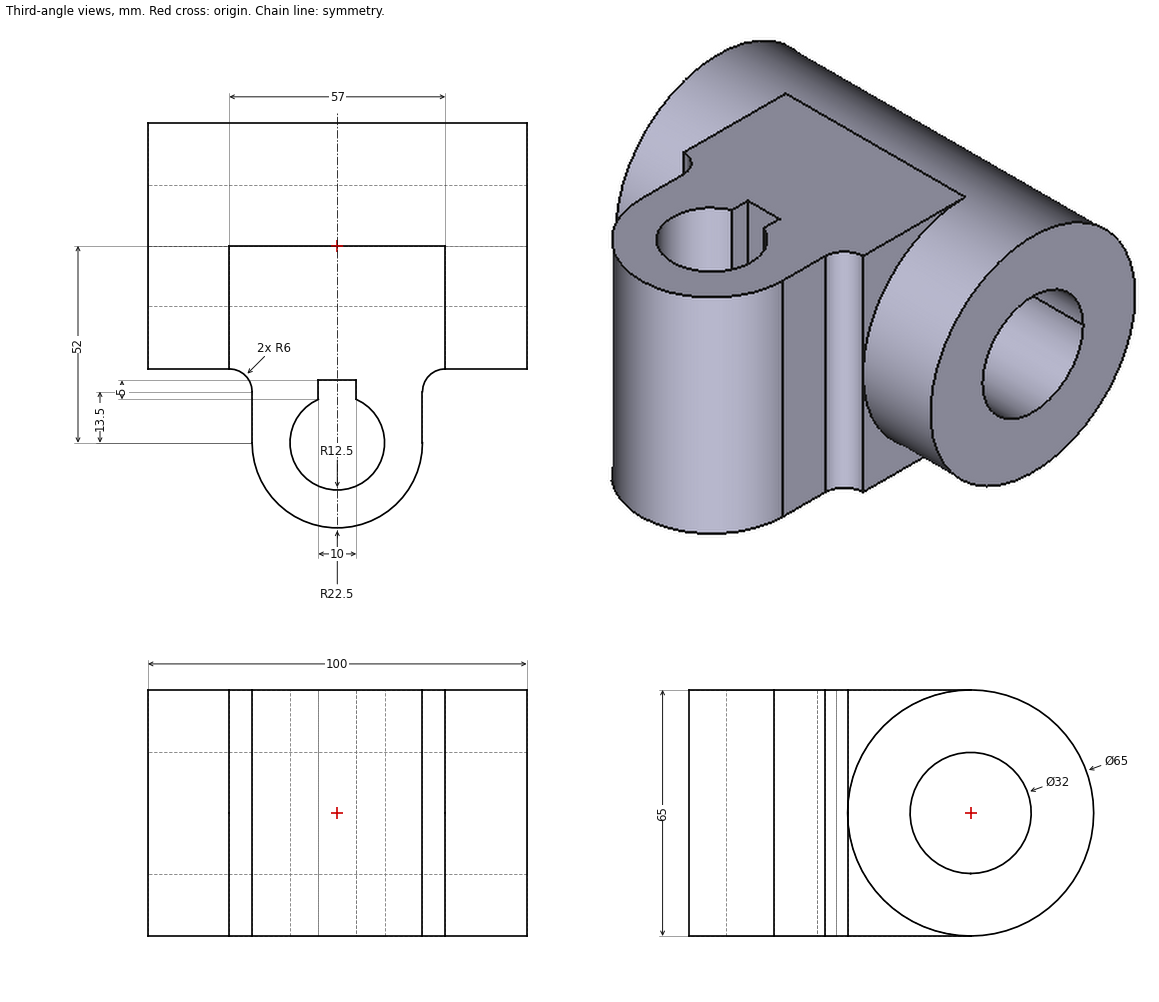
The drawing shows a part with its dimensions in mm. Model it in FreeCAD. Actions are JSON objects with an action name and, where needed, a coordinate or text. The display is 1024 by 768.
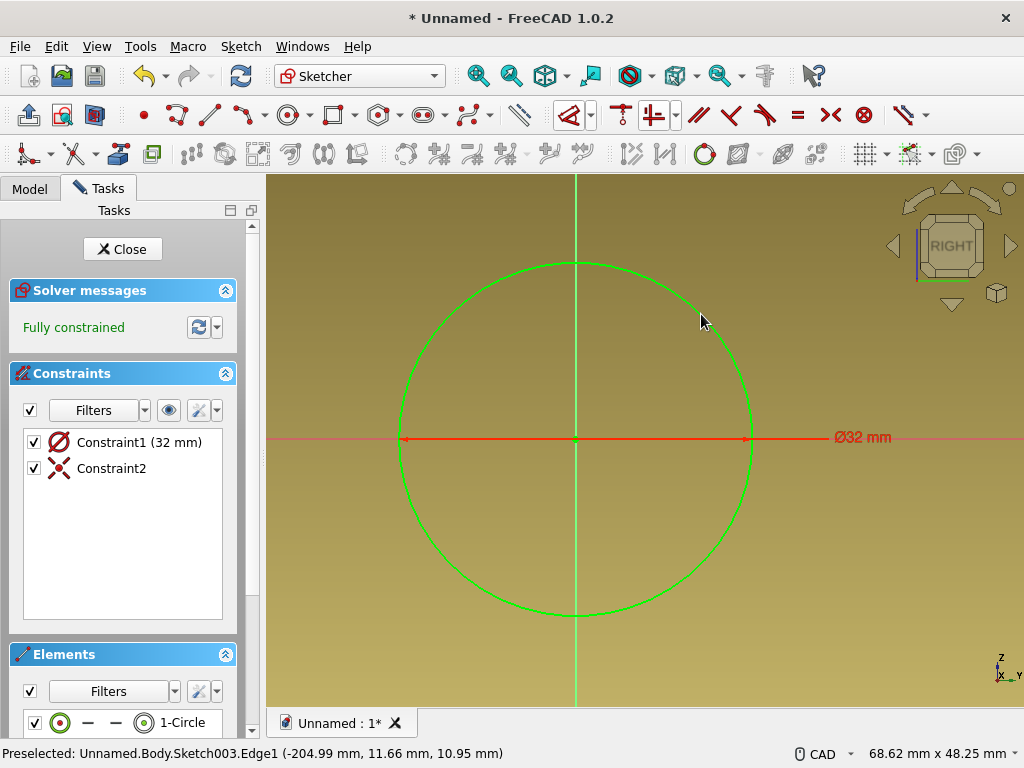
{"action": "left_click", "coordinate": [123, 249]}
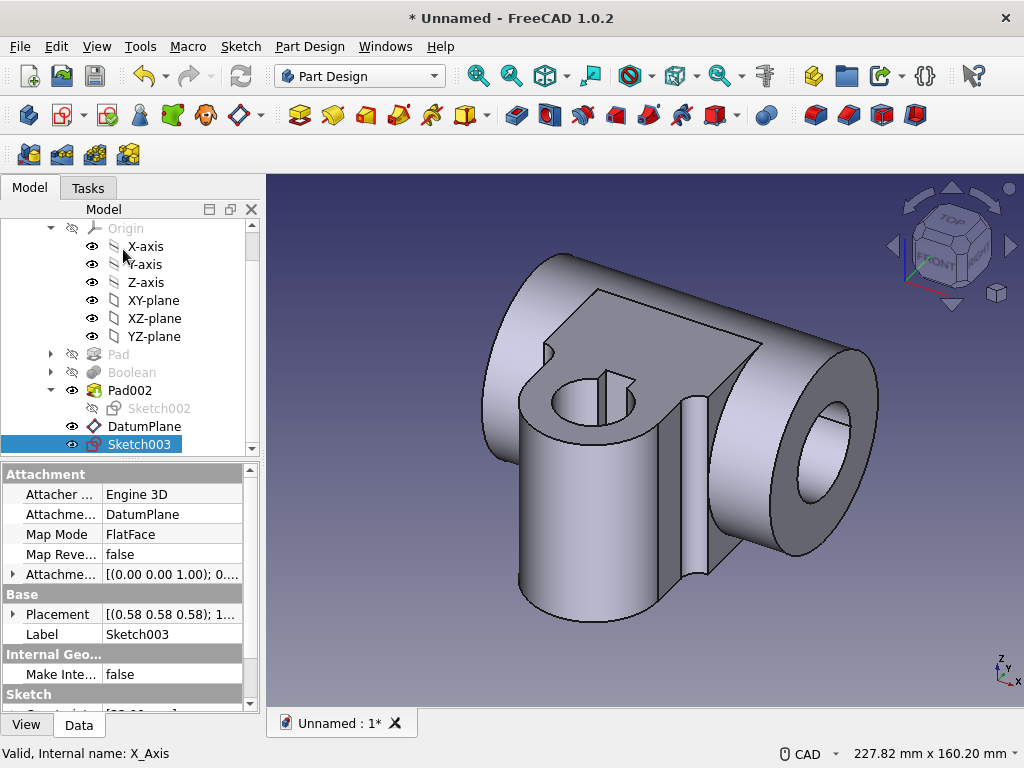
{"action": "left_click", "coordinate": [517, 116]}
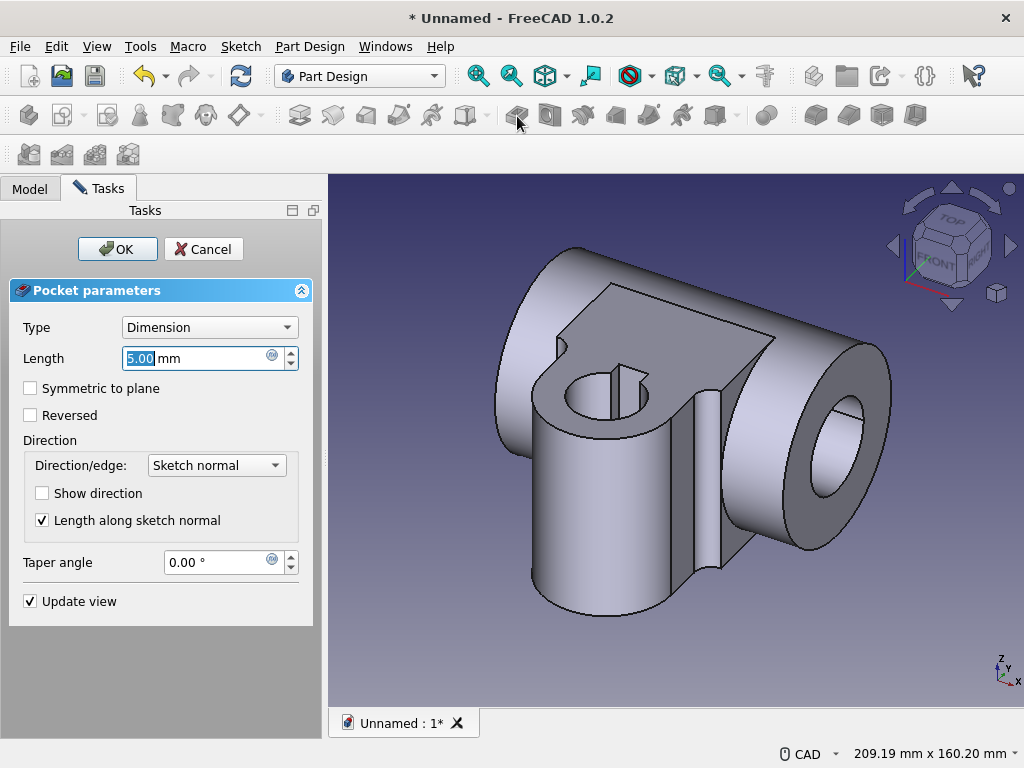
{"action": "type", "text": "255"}
{"action": "key", "text": "Tab"}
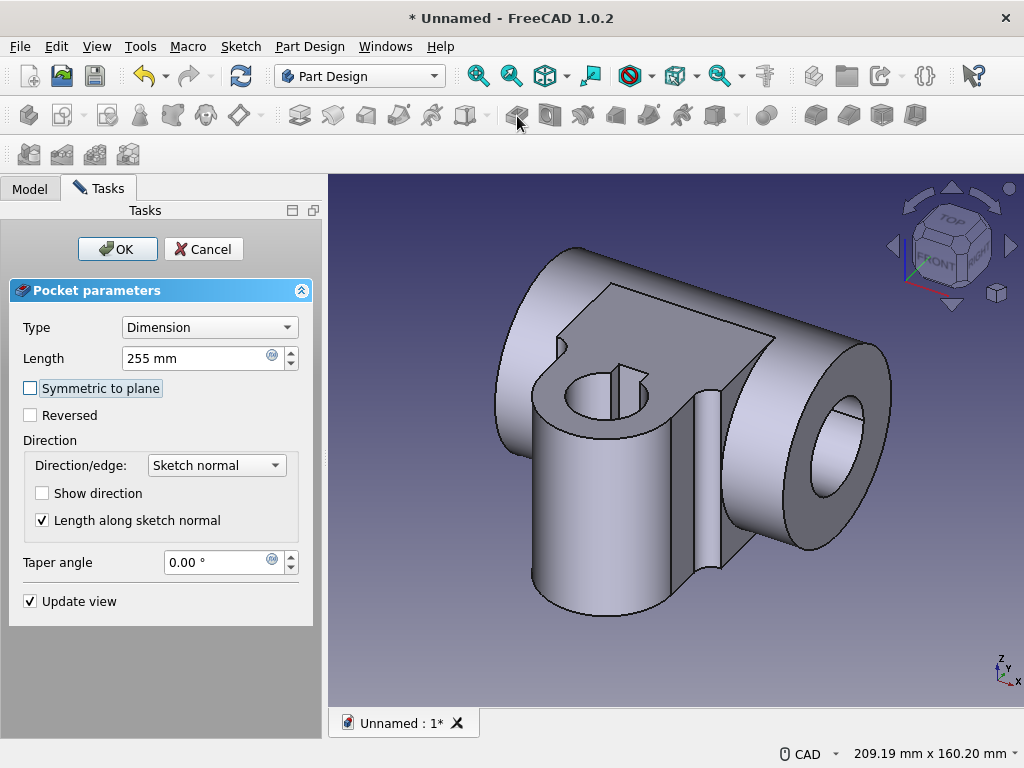
{"action": "left_click", "coordinate": [31, 415]}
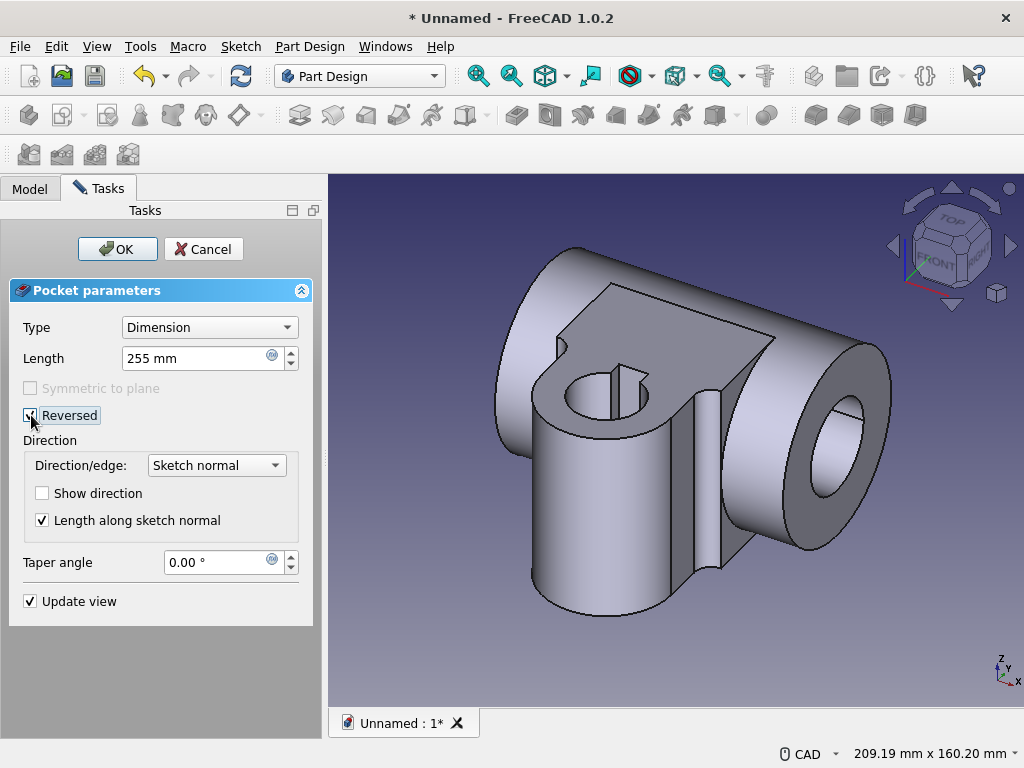
{"action": "left_click", "coordinate": [118, 249]}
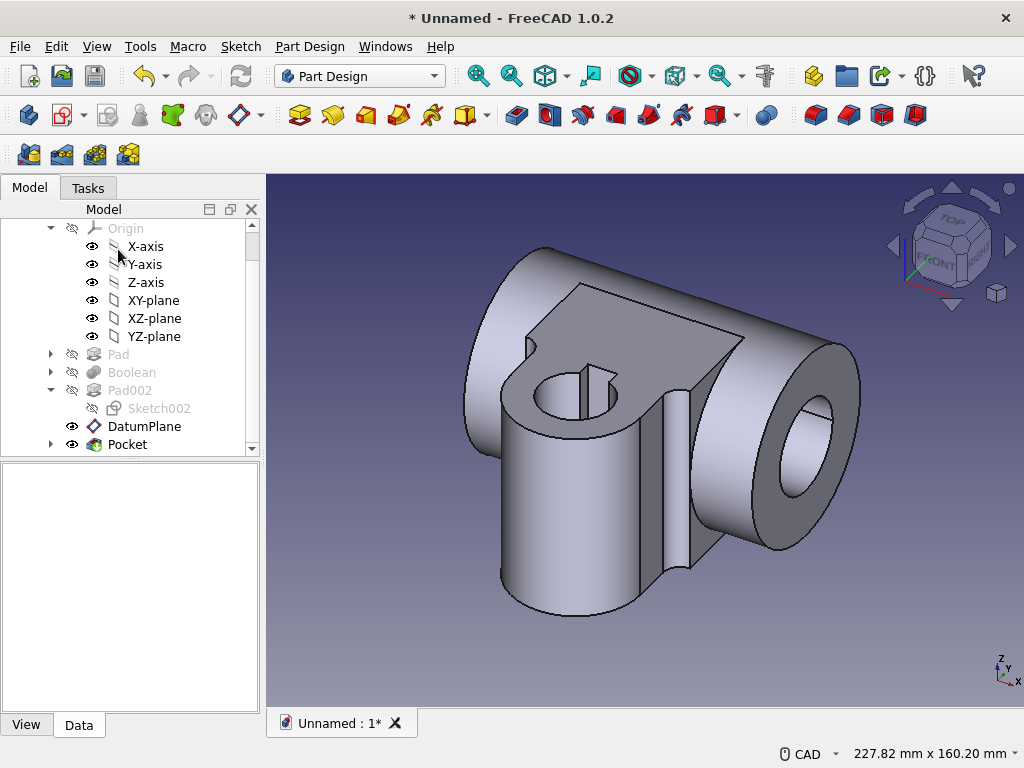
{"action": "left_click", "coordinate": [117, 426]}
{"action": "key", "text": "space"}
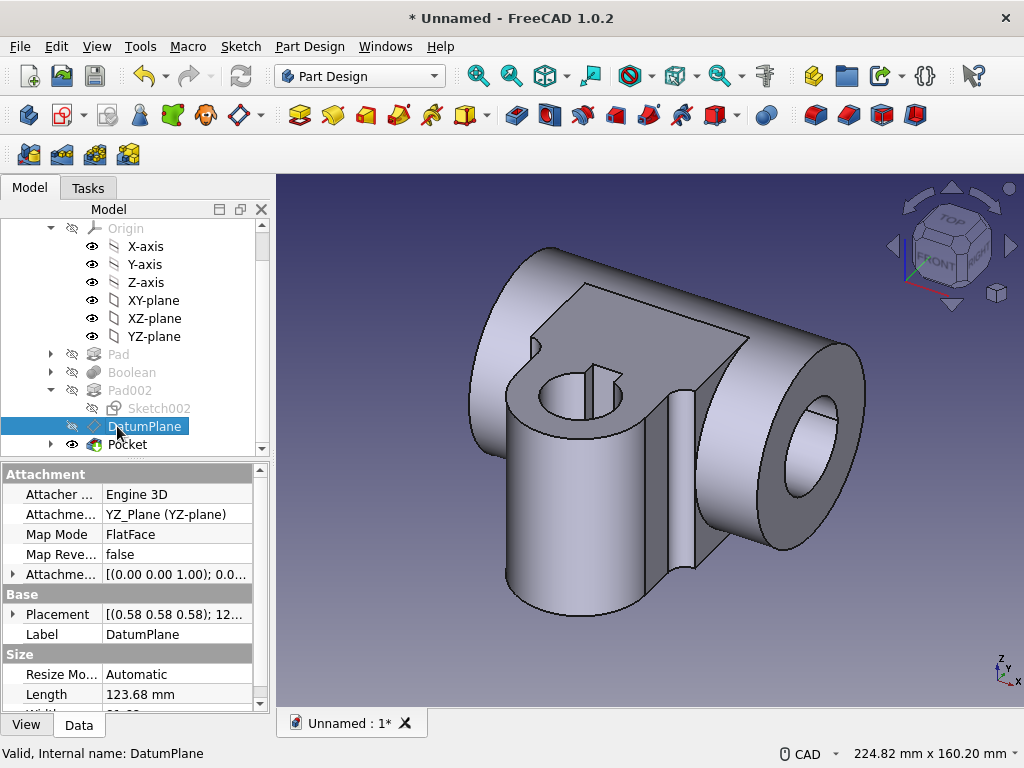
{"action": "key", "text": "0"}